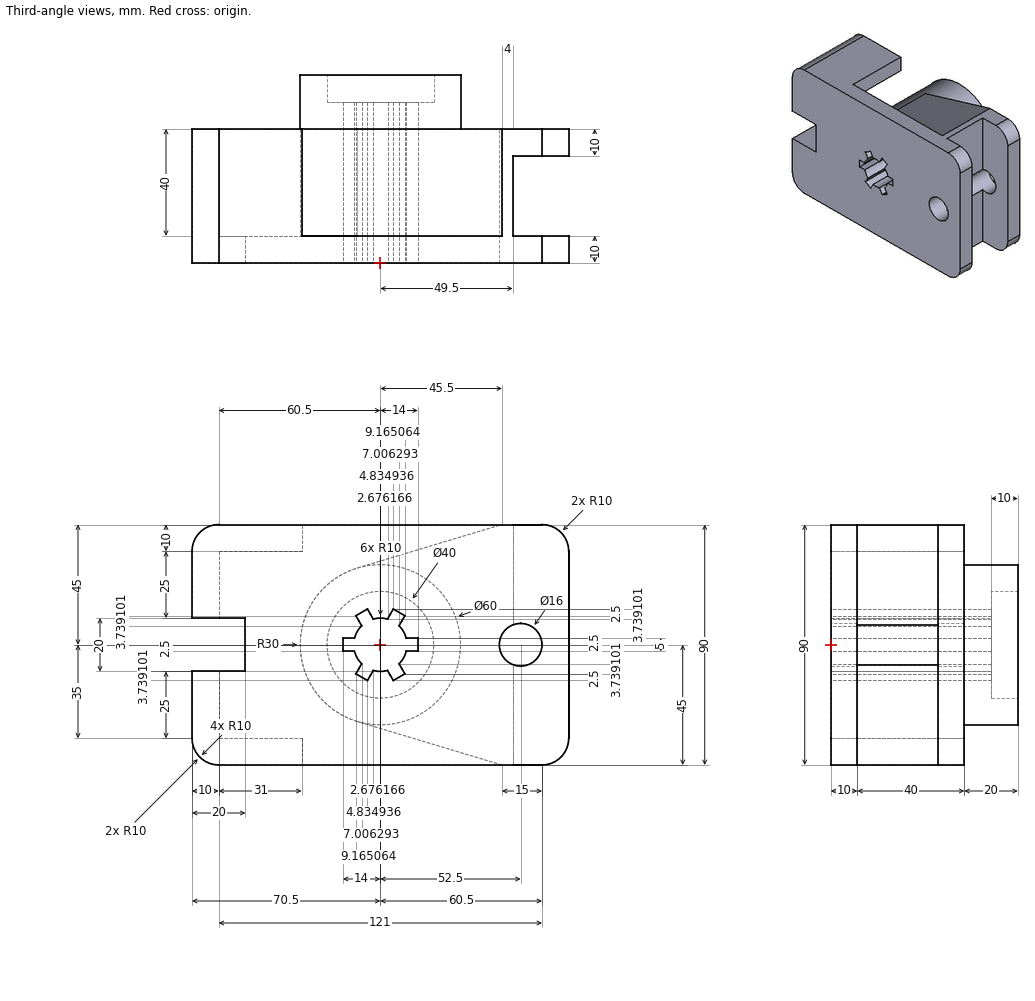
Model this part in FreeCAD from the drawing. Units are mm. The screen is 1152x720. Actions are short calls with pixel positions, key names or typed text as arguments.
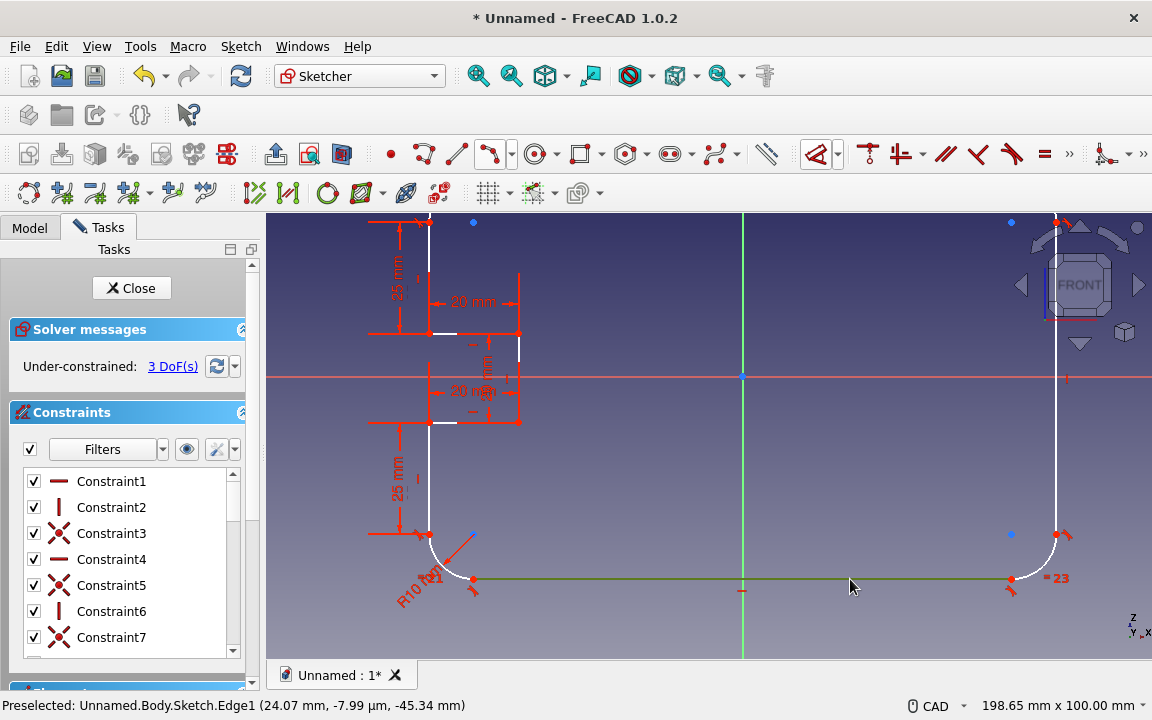
click(838, 154)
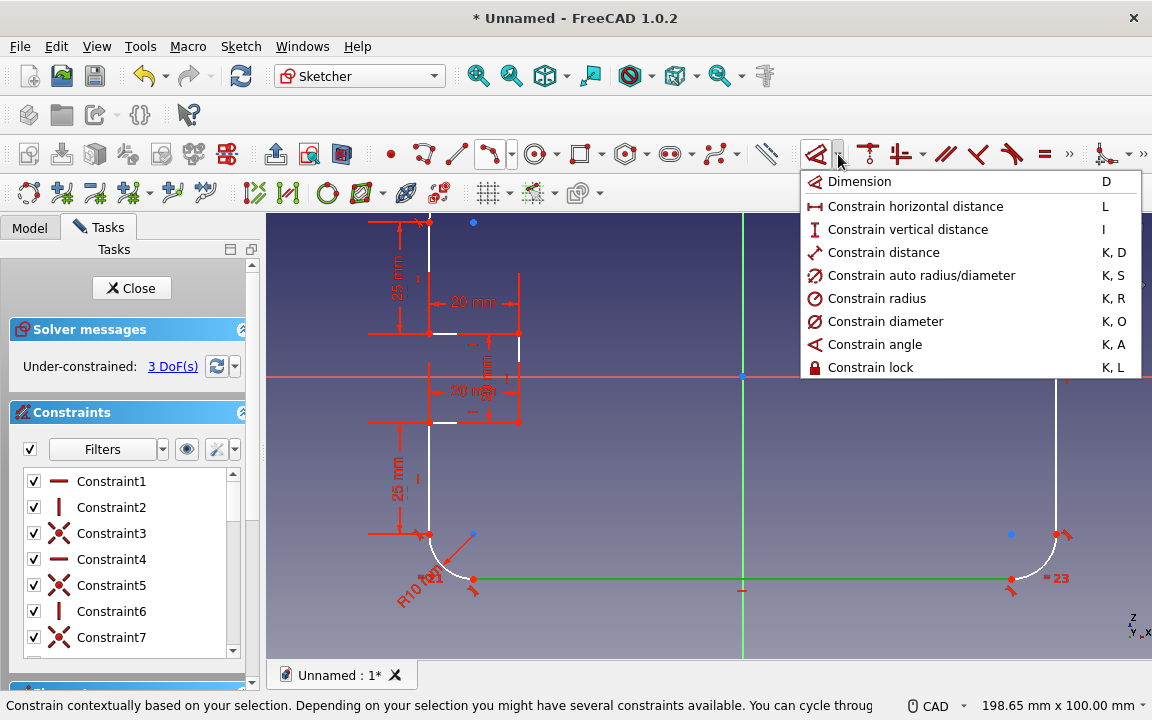
click(971, 206)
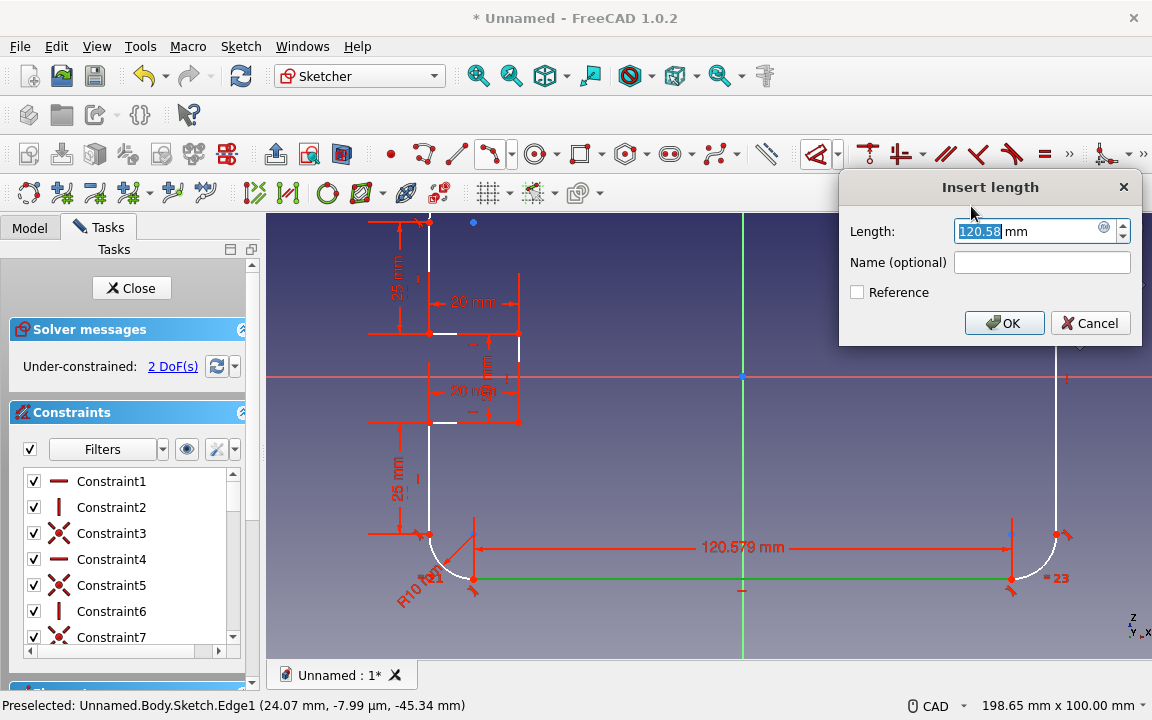
text(121)
key(Return)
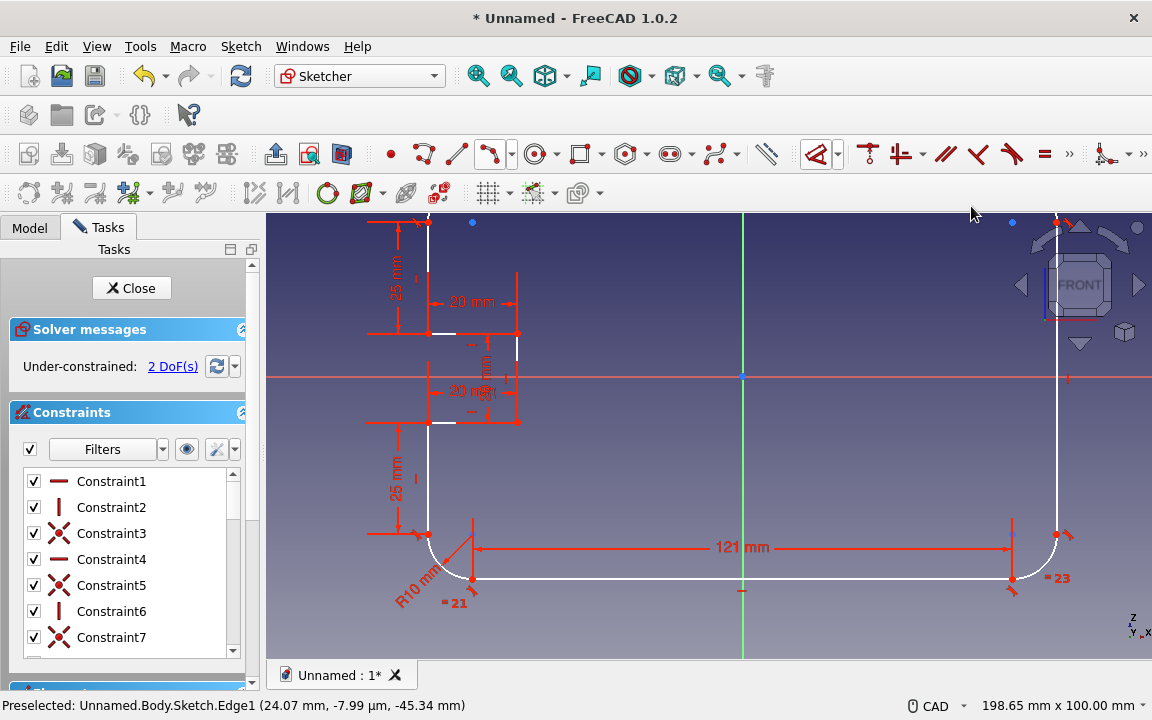
scroll(433, 556, down, 2)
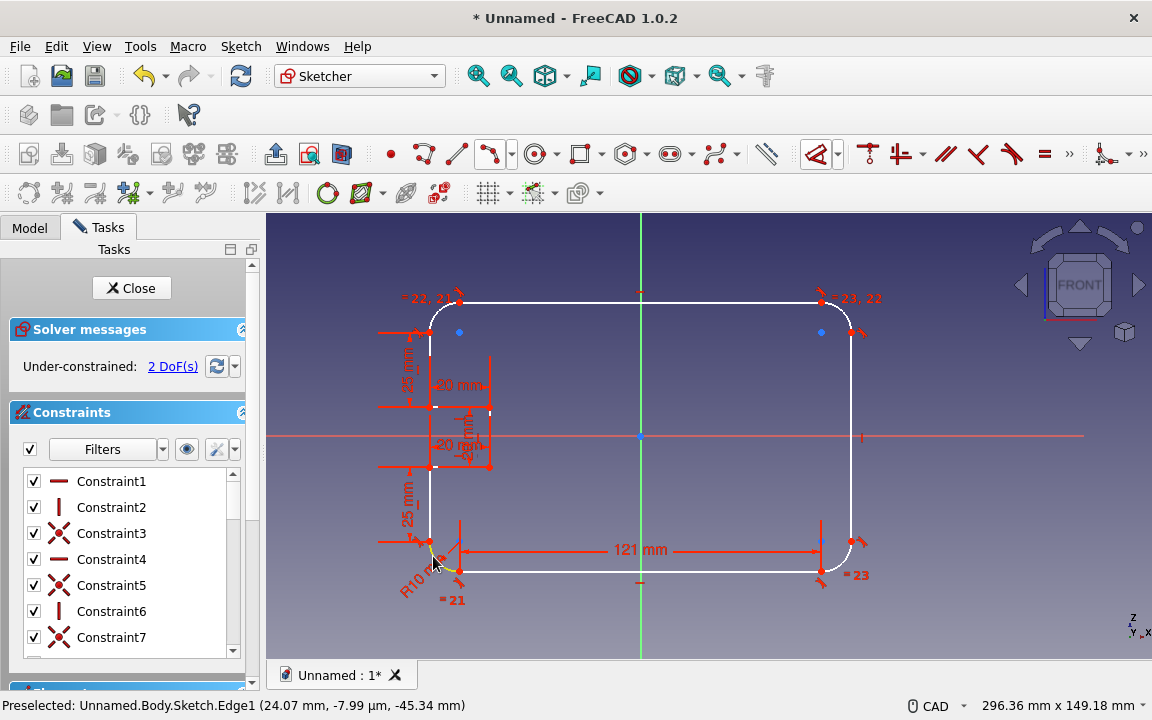
click(821, 572)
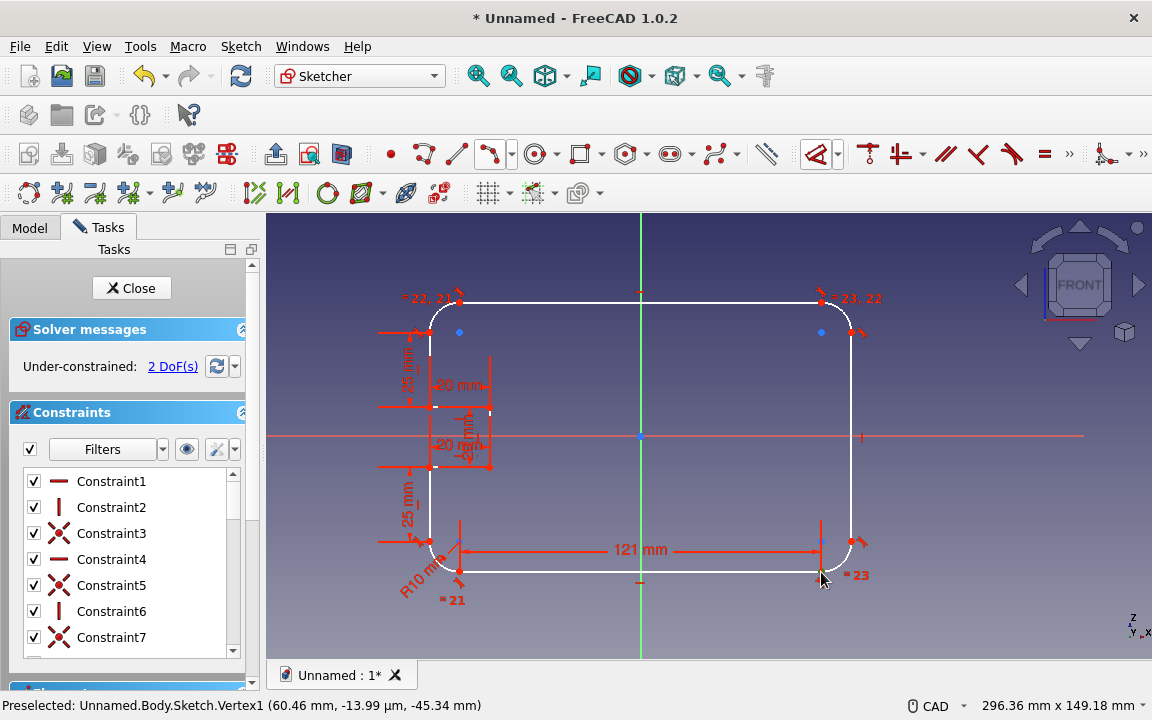
click(838, 154)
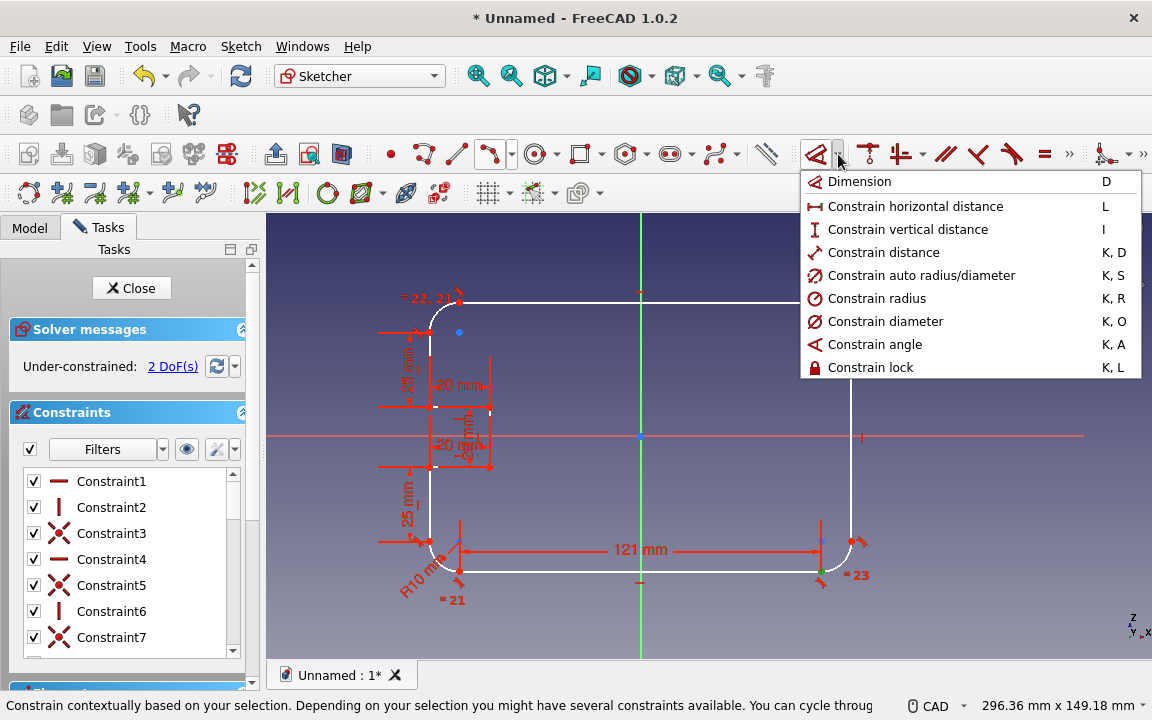
click(971, 230)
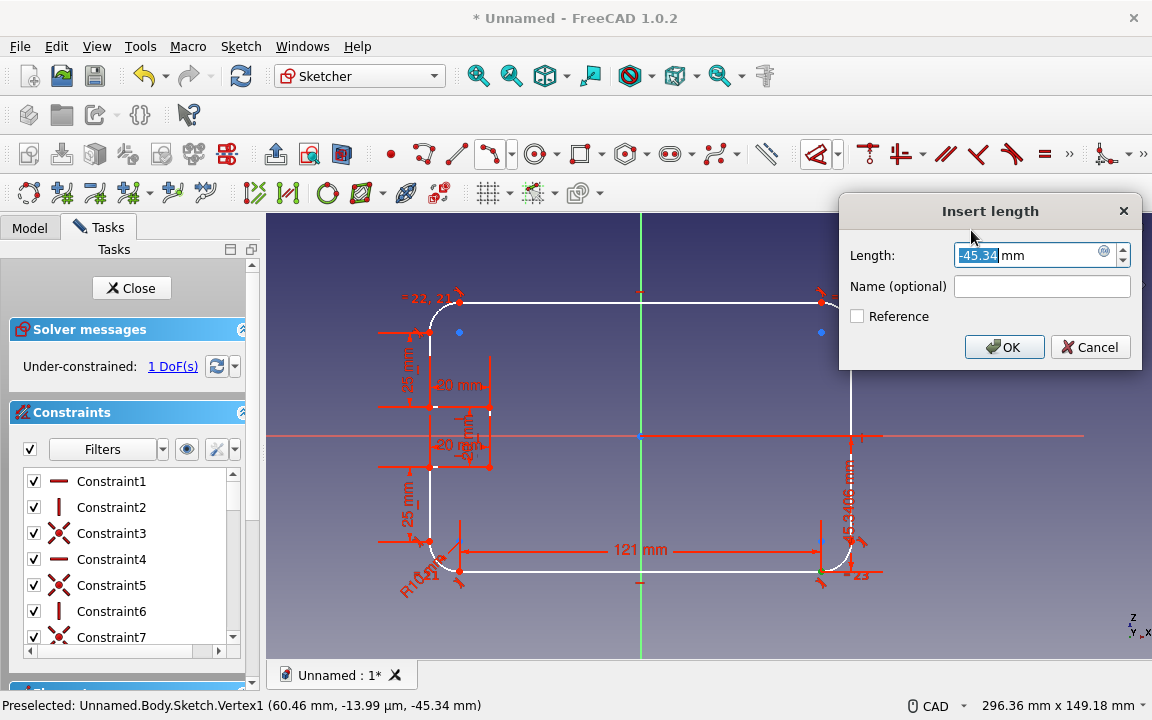
text(-45)
key(Return)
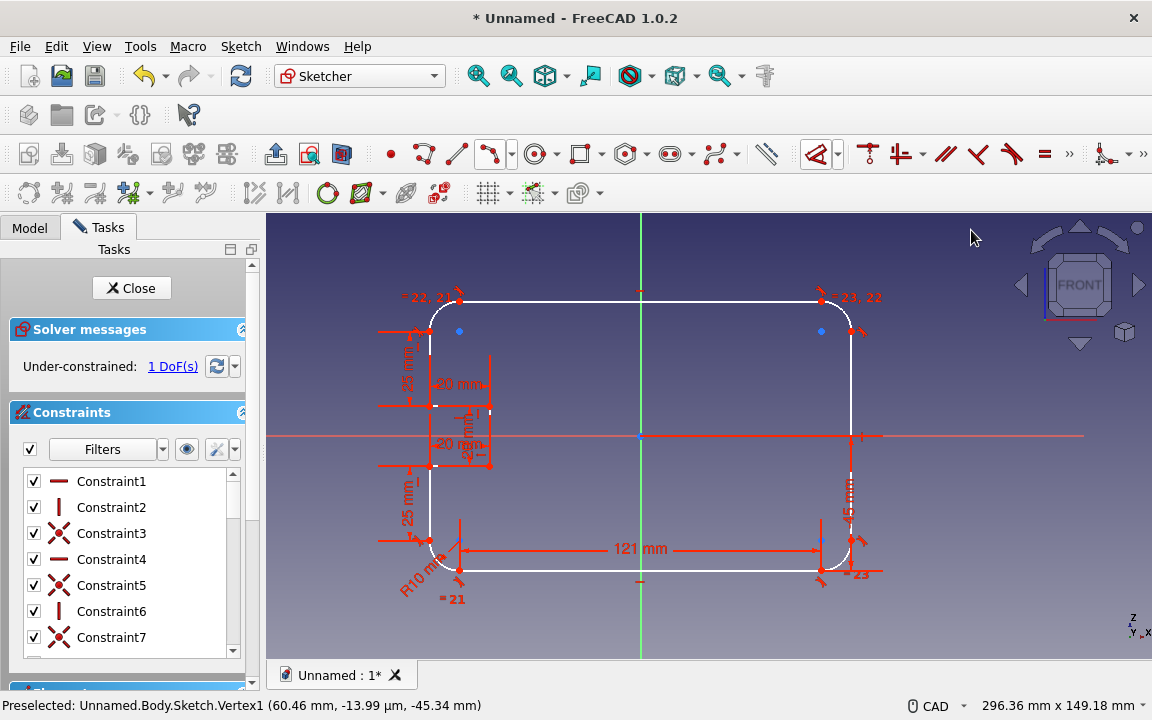
click(821, 571)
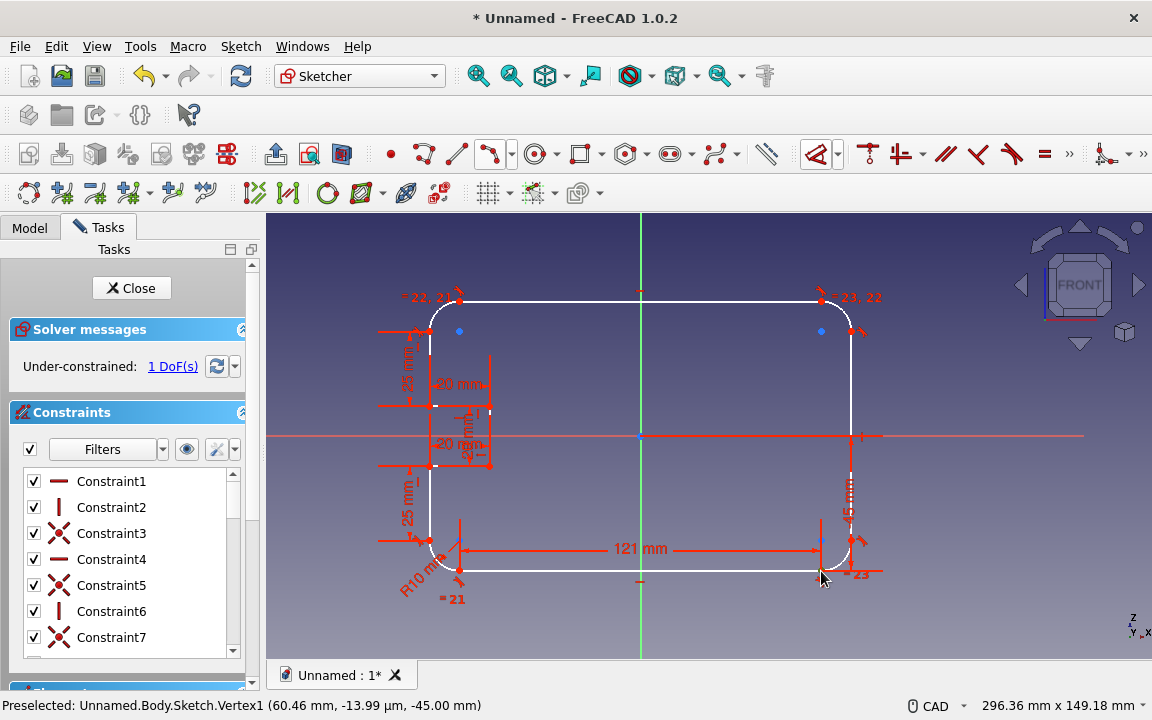
key(l)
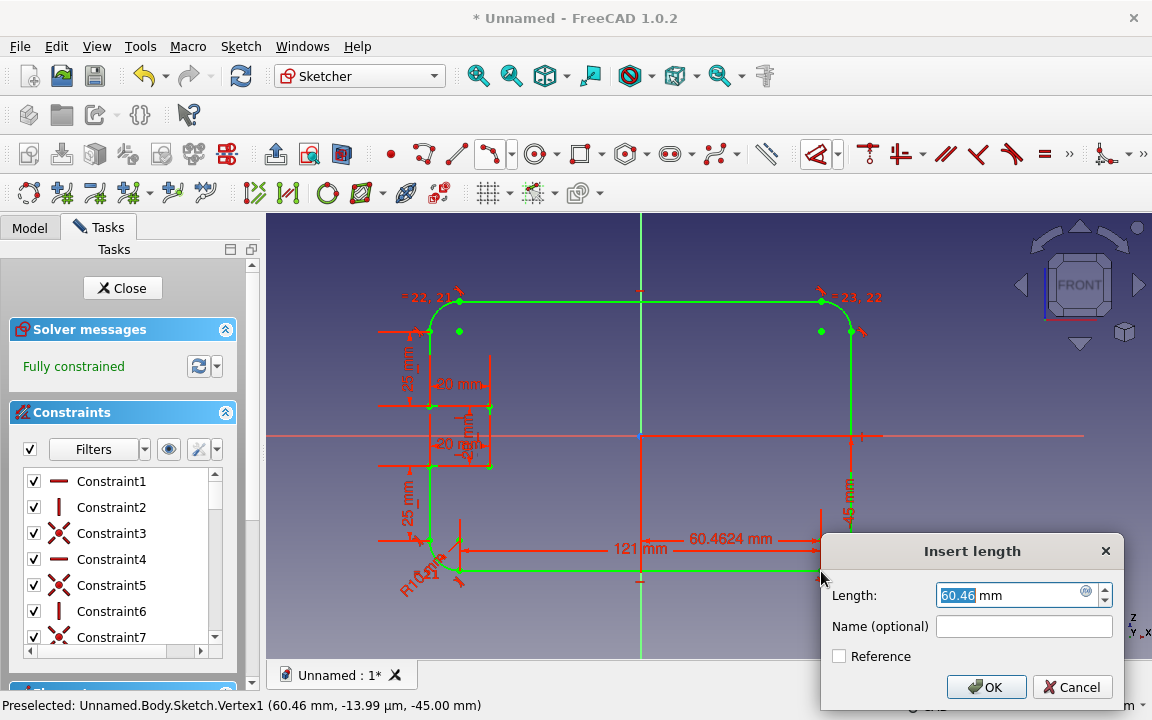
text(60.5)
key(Return)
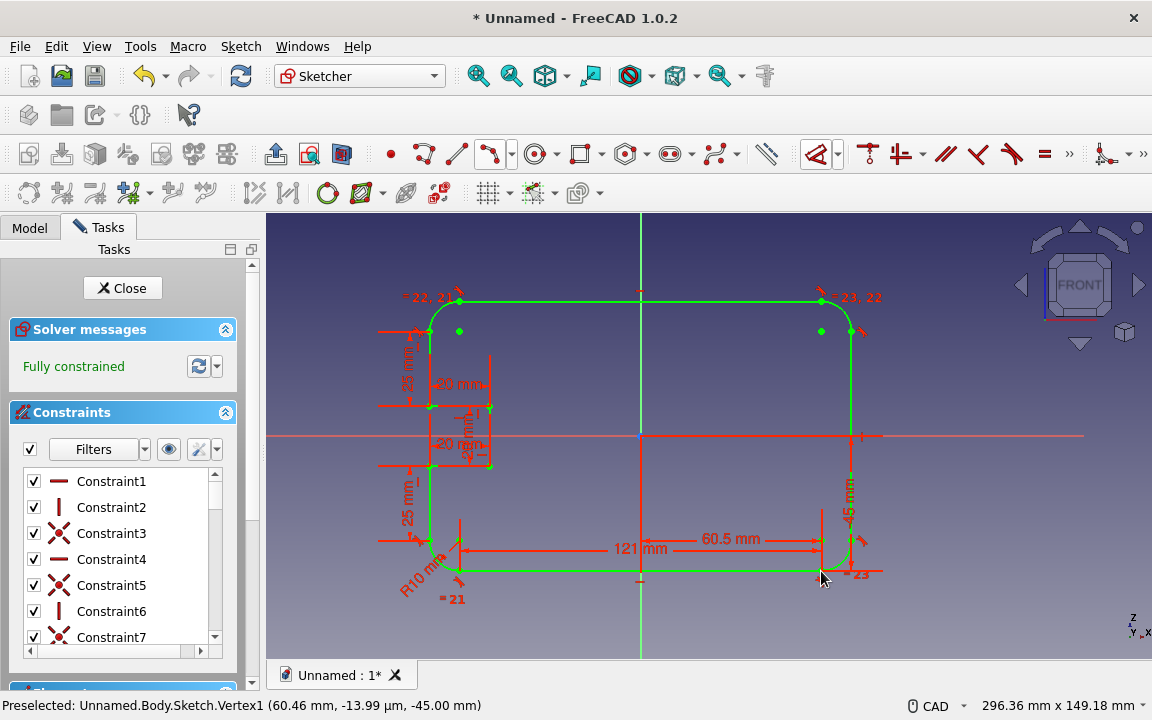
click(123, 288)